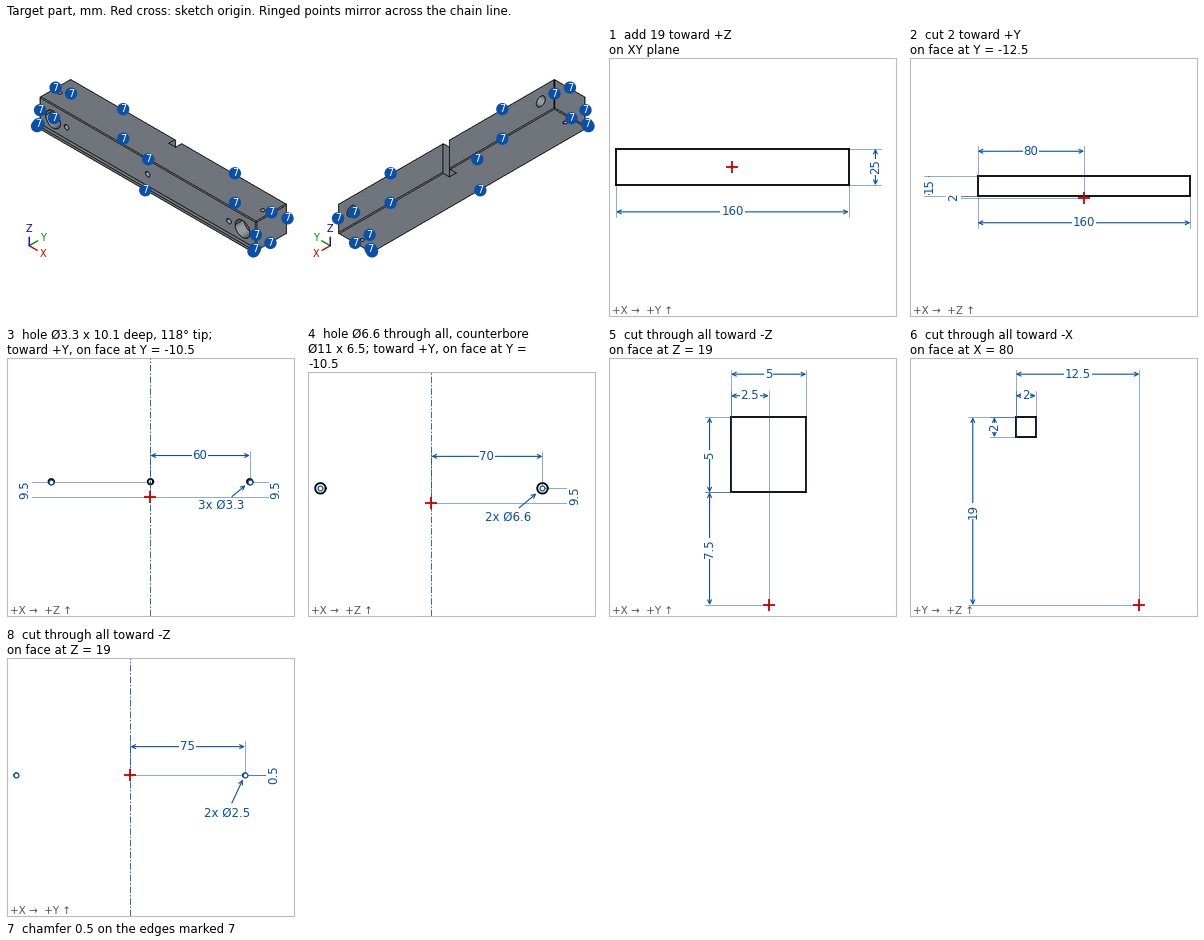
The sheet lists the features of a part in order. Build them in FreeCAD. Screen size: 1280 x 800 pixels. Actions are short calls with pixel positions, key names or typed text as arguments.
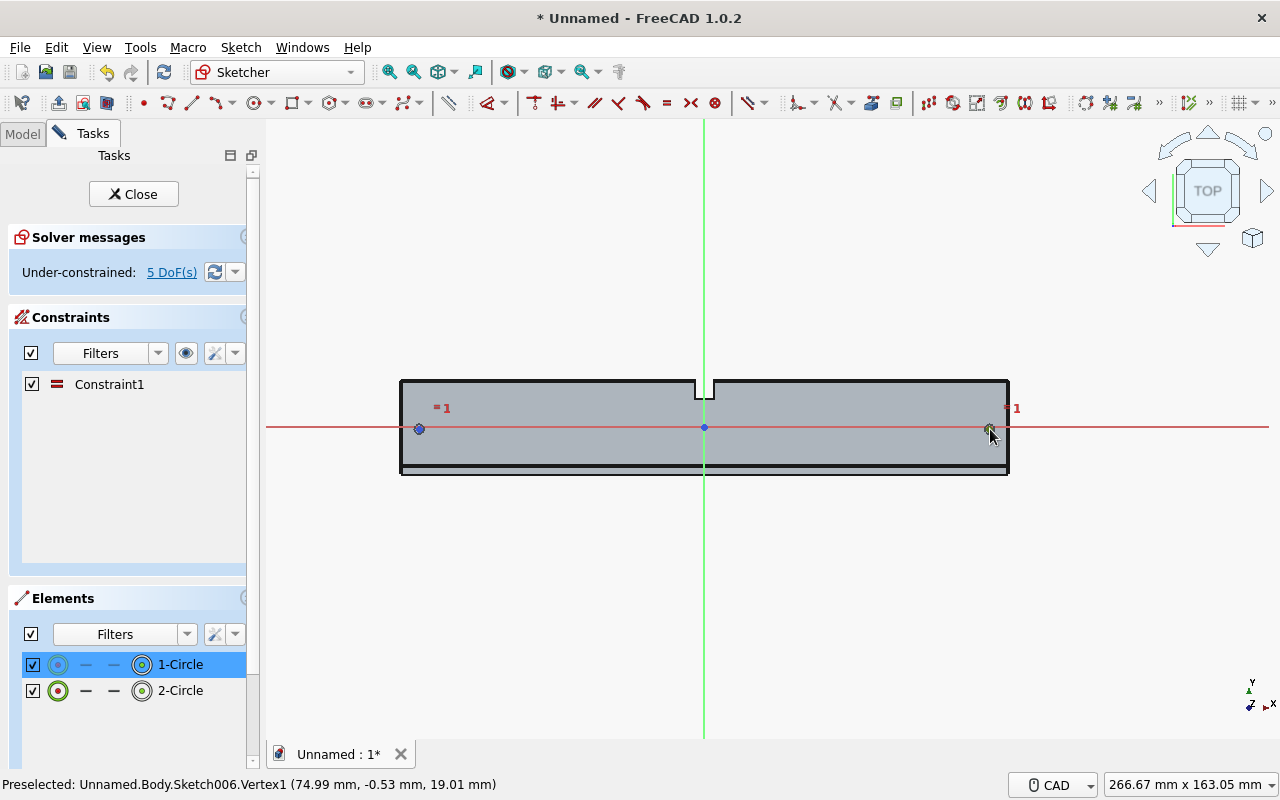
click(419, 429)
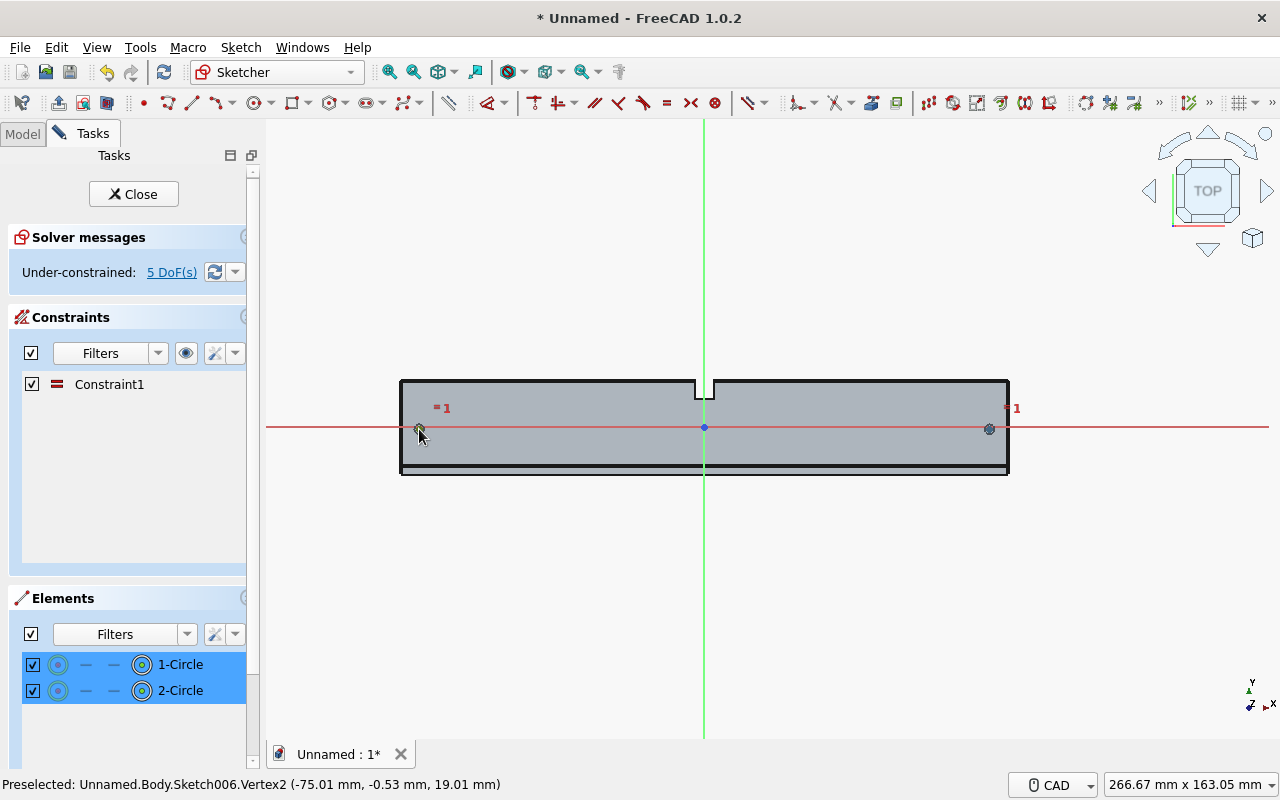
click(704, 671)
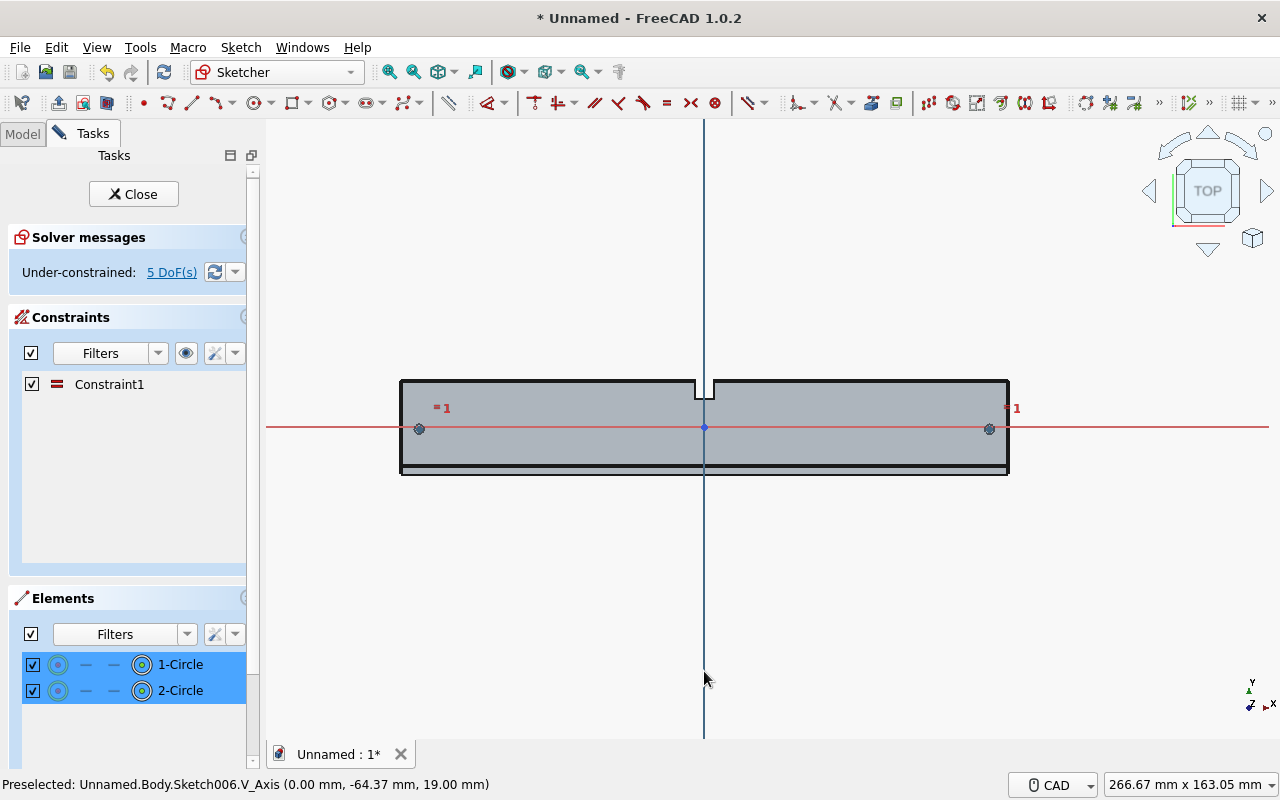
click(692, 104)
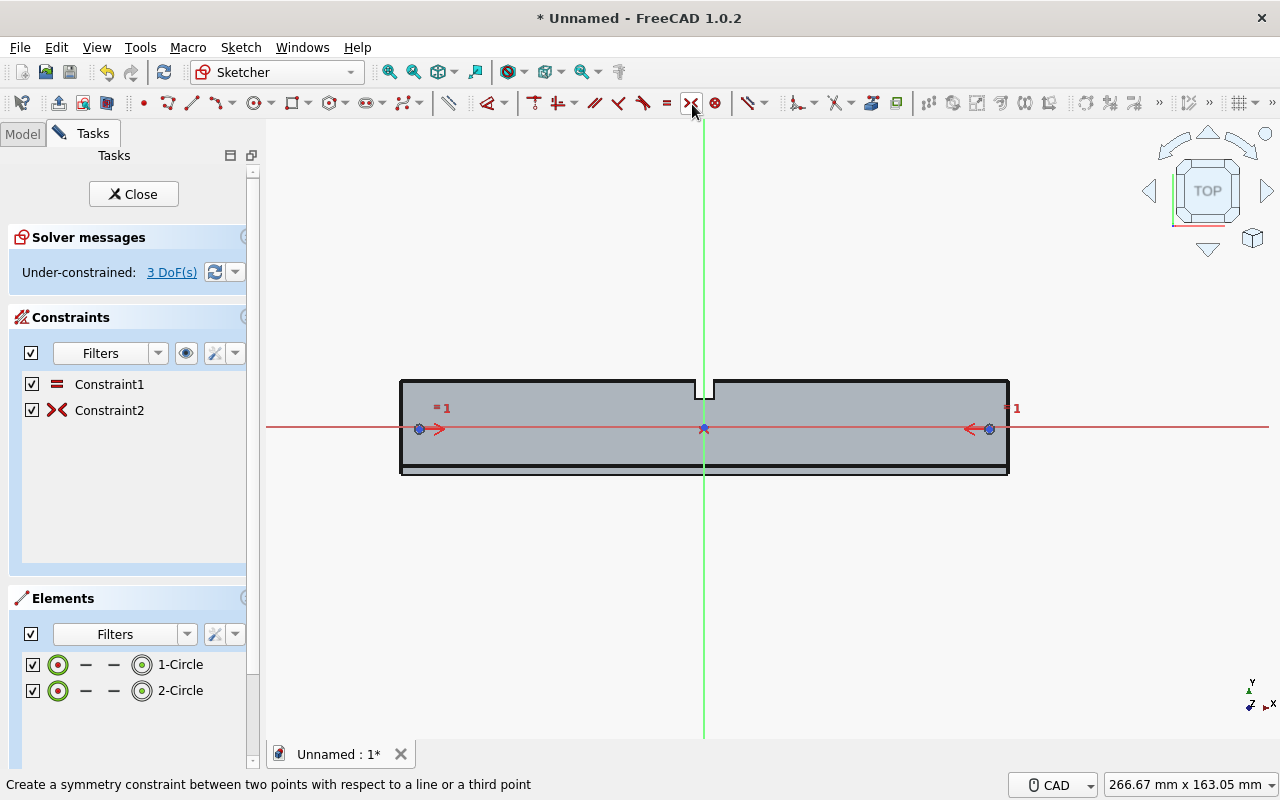
click(488, 104)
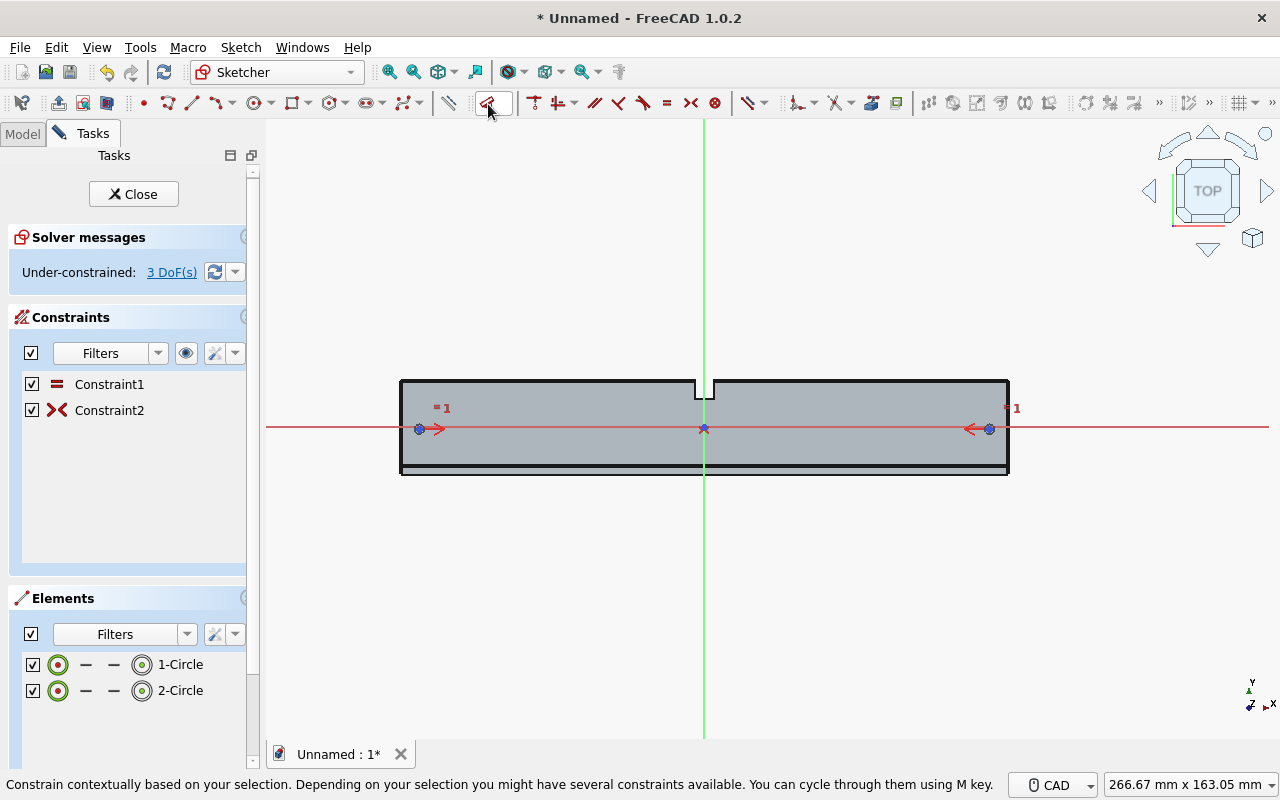
scroll(993, 433, up, 8)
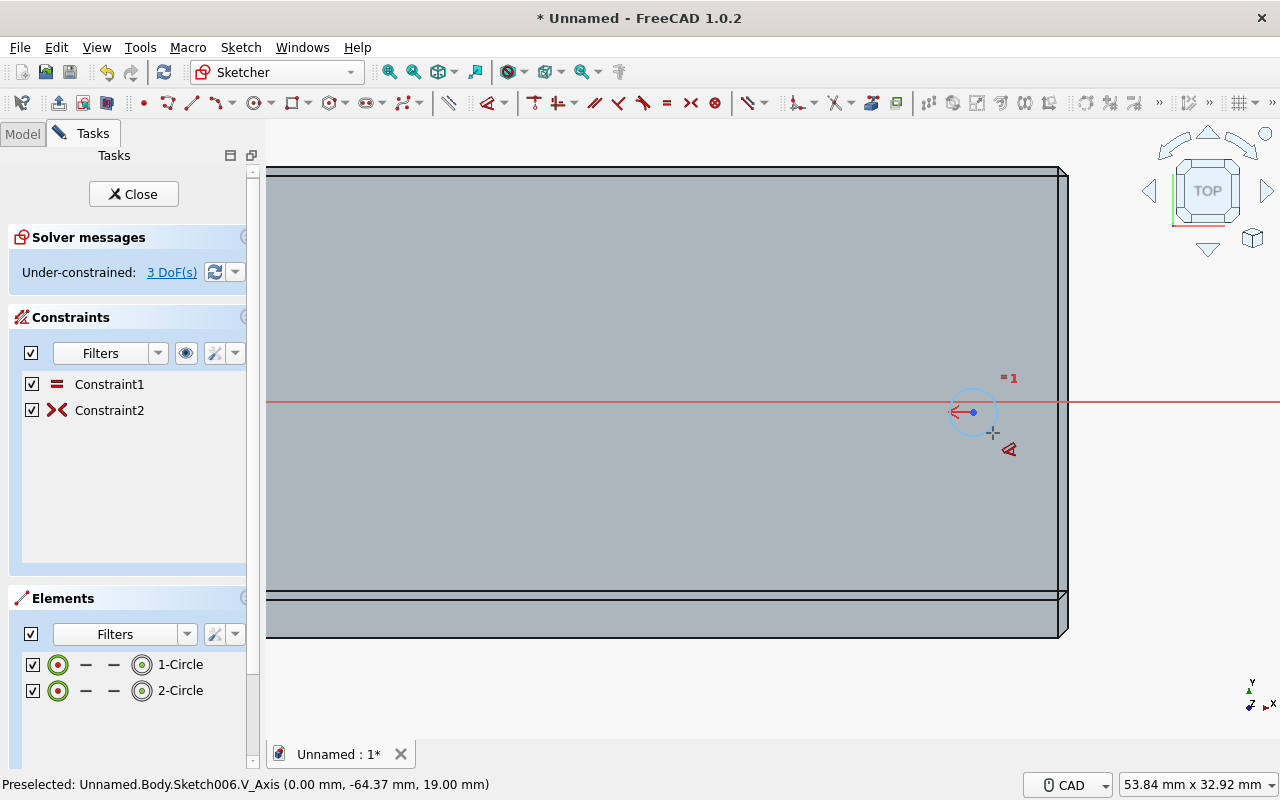
click(990, 429)
click(1013, 452)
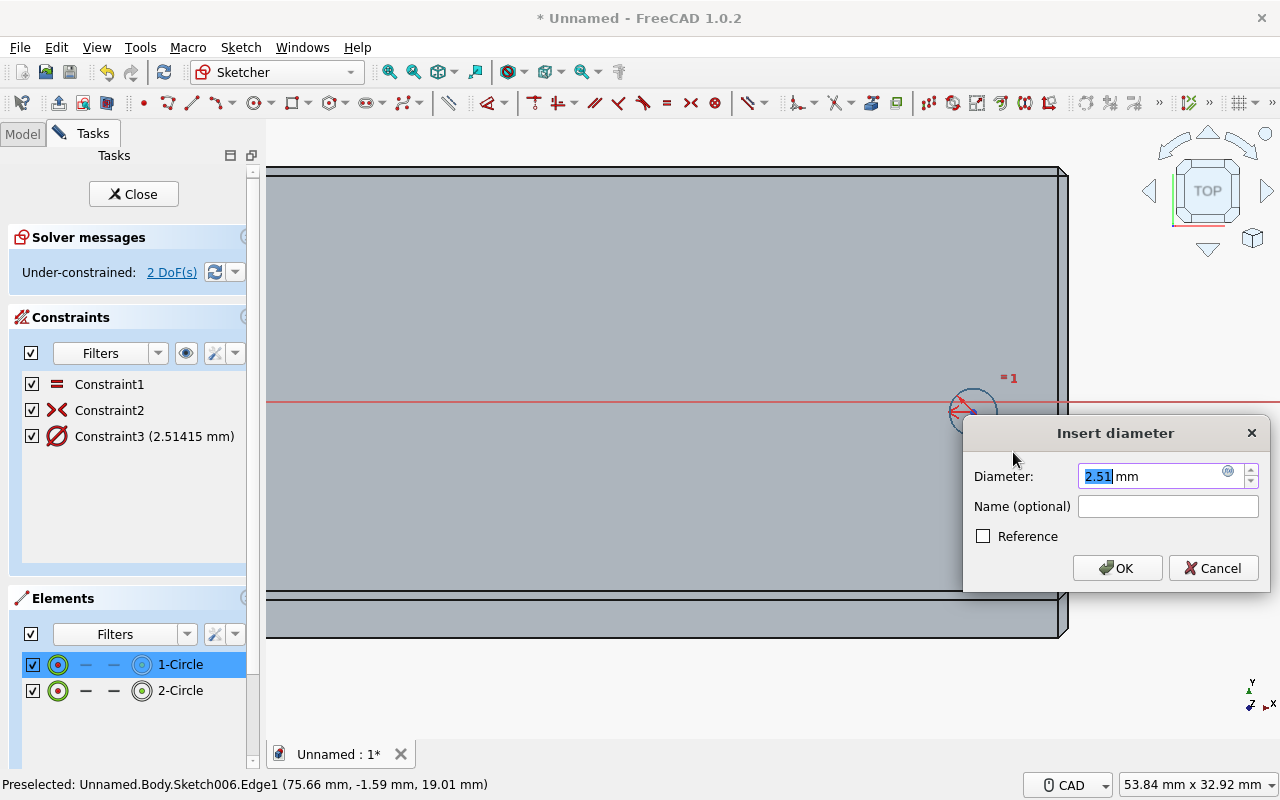
text(2.5)
key(Return)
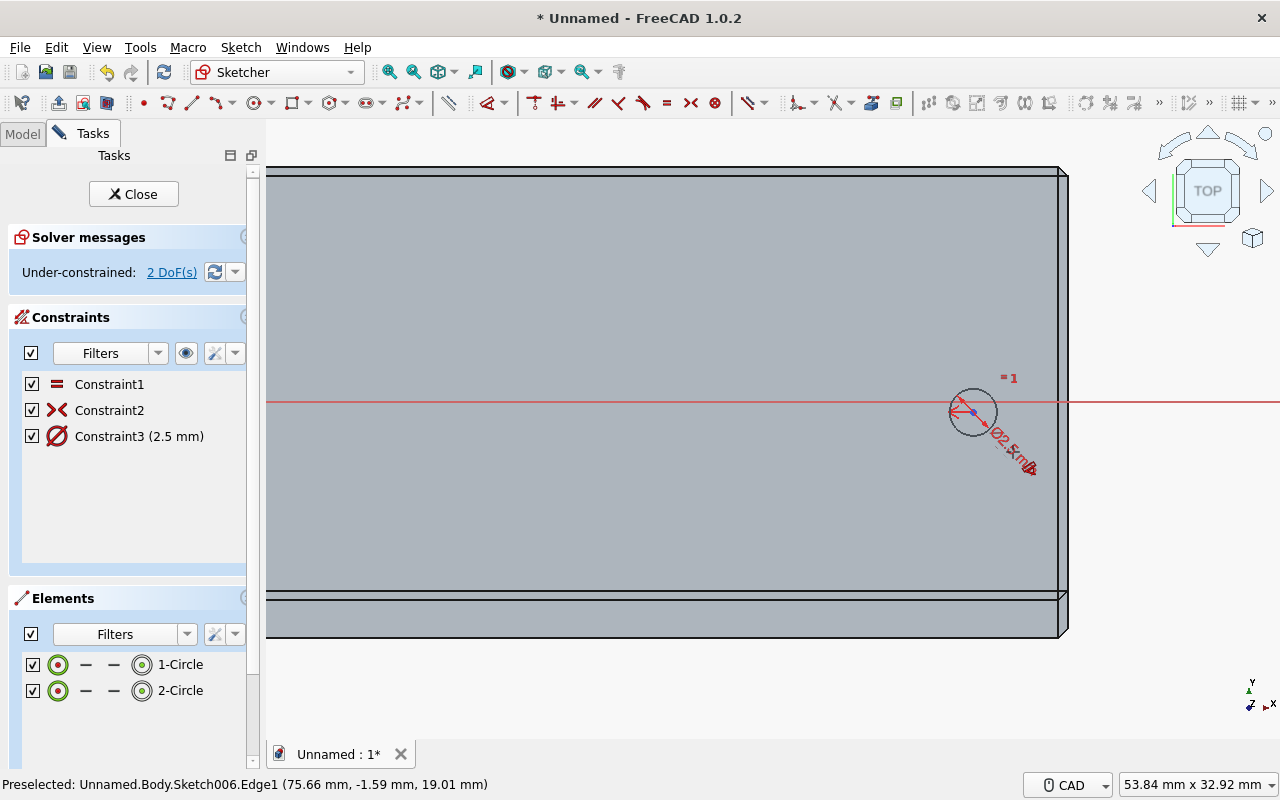
scroll(994, 433, down, 8)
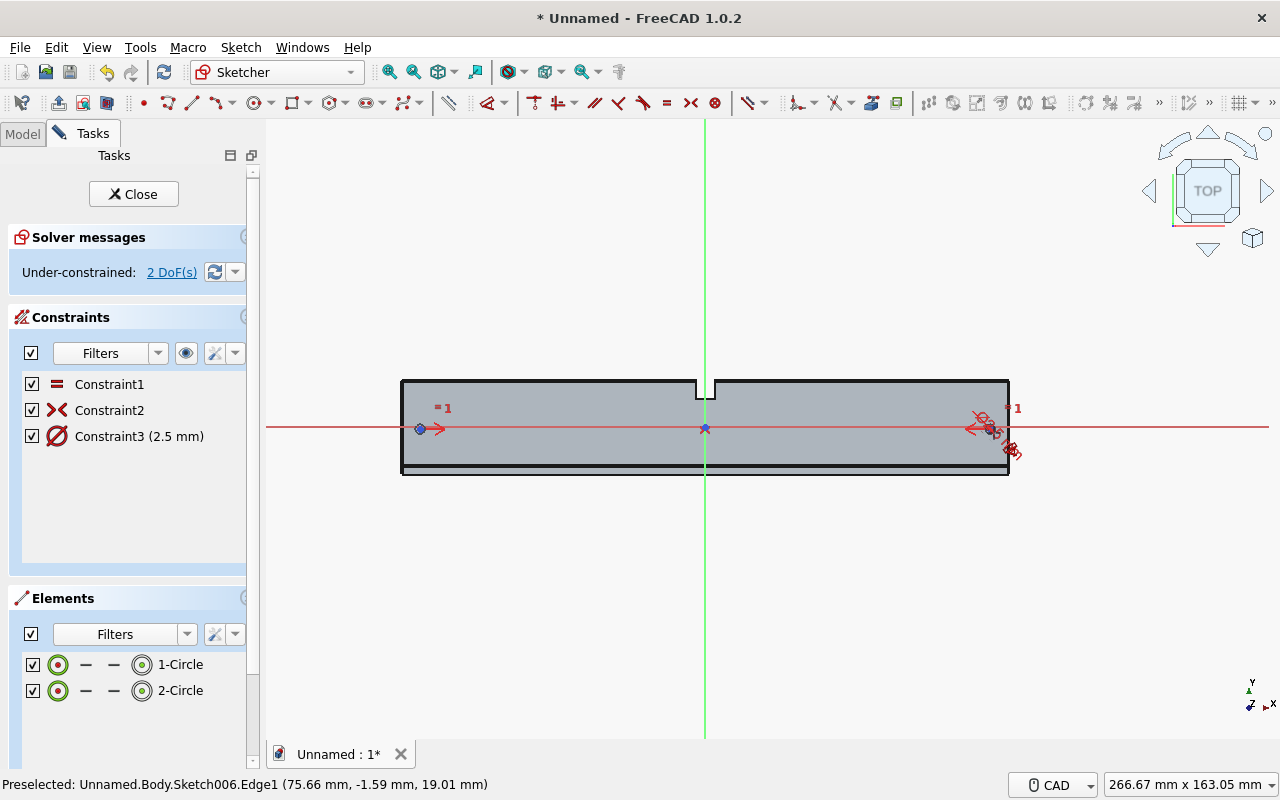
click(990, 429)
click(848, 393)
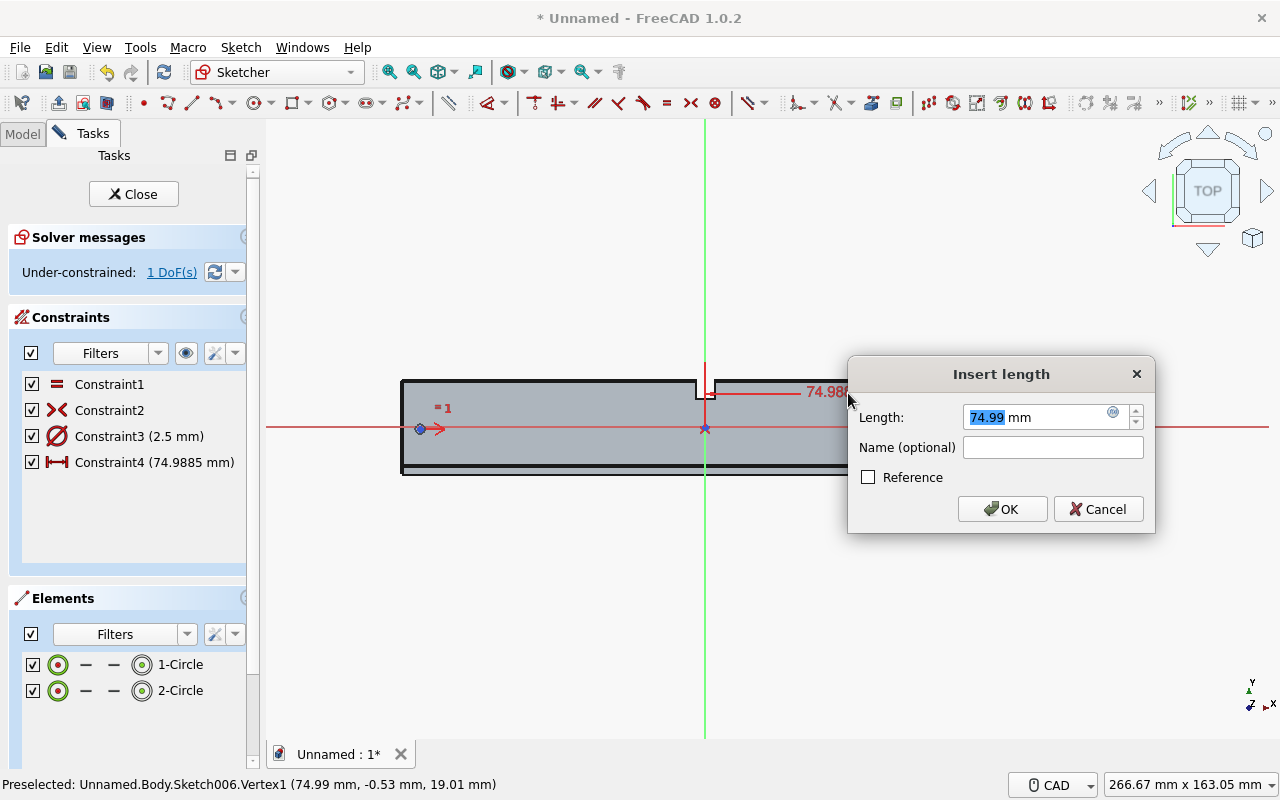
text(75)
key(Return)